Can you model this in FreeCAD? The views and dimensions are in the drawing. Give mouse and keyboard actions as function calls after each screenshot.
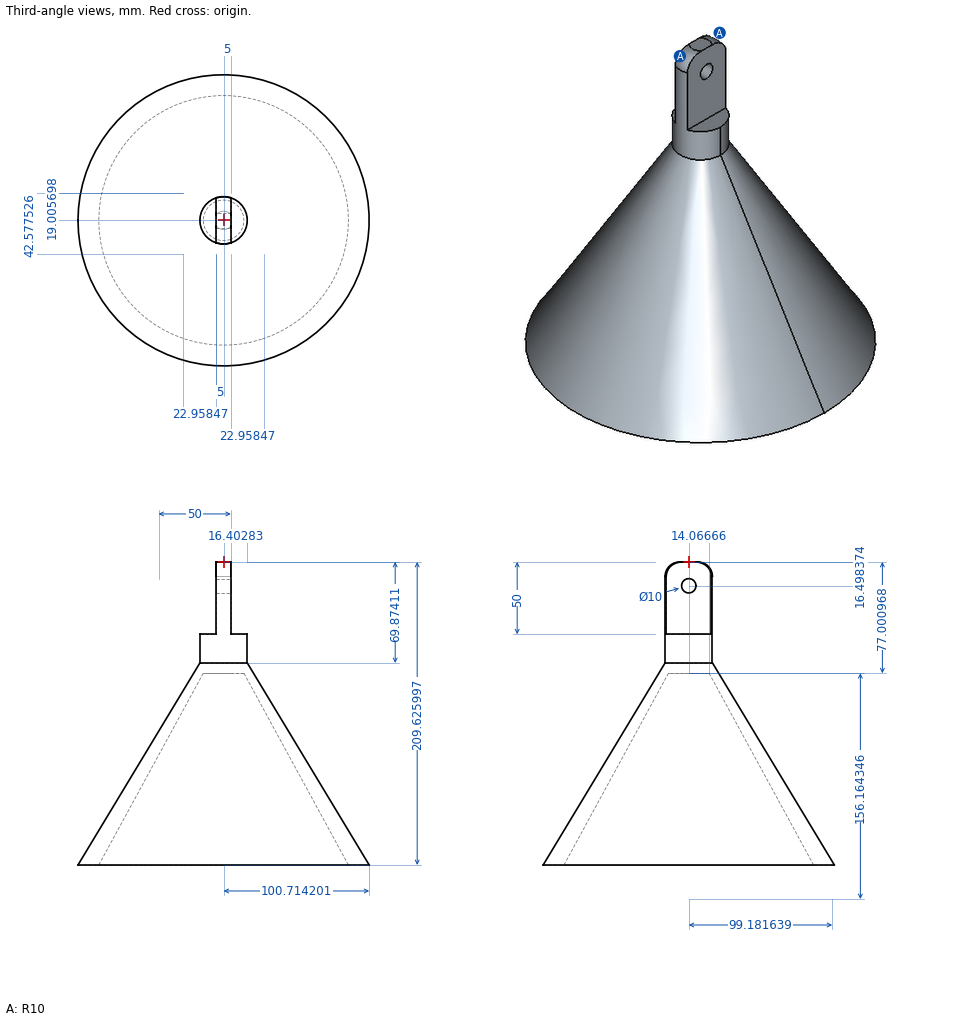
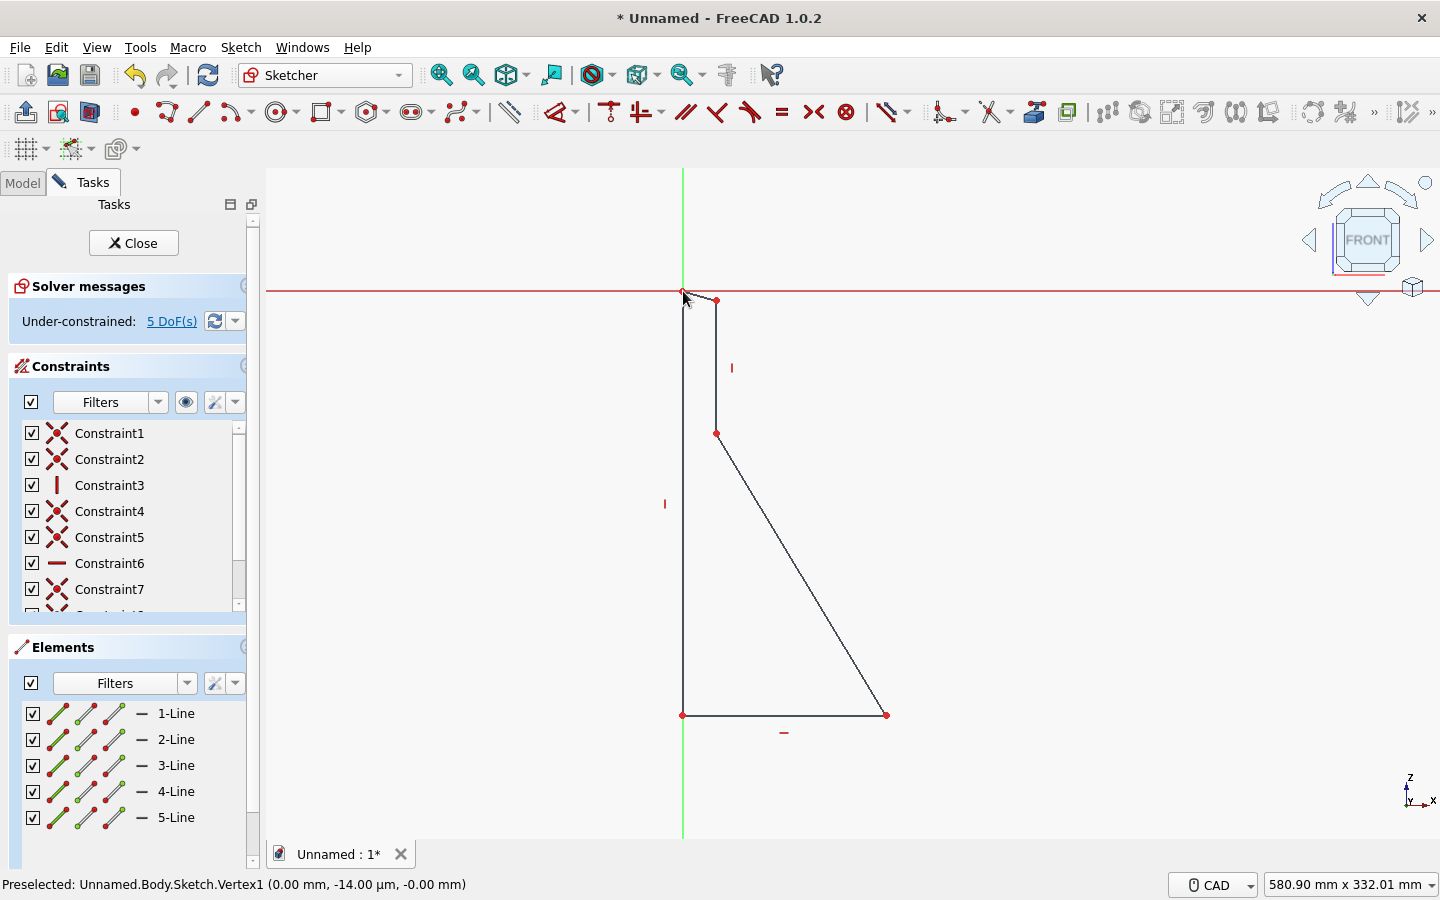
scroll(693, 294, up, 2)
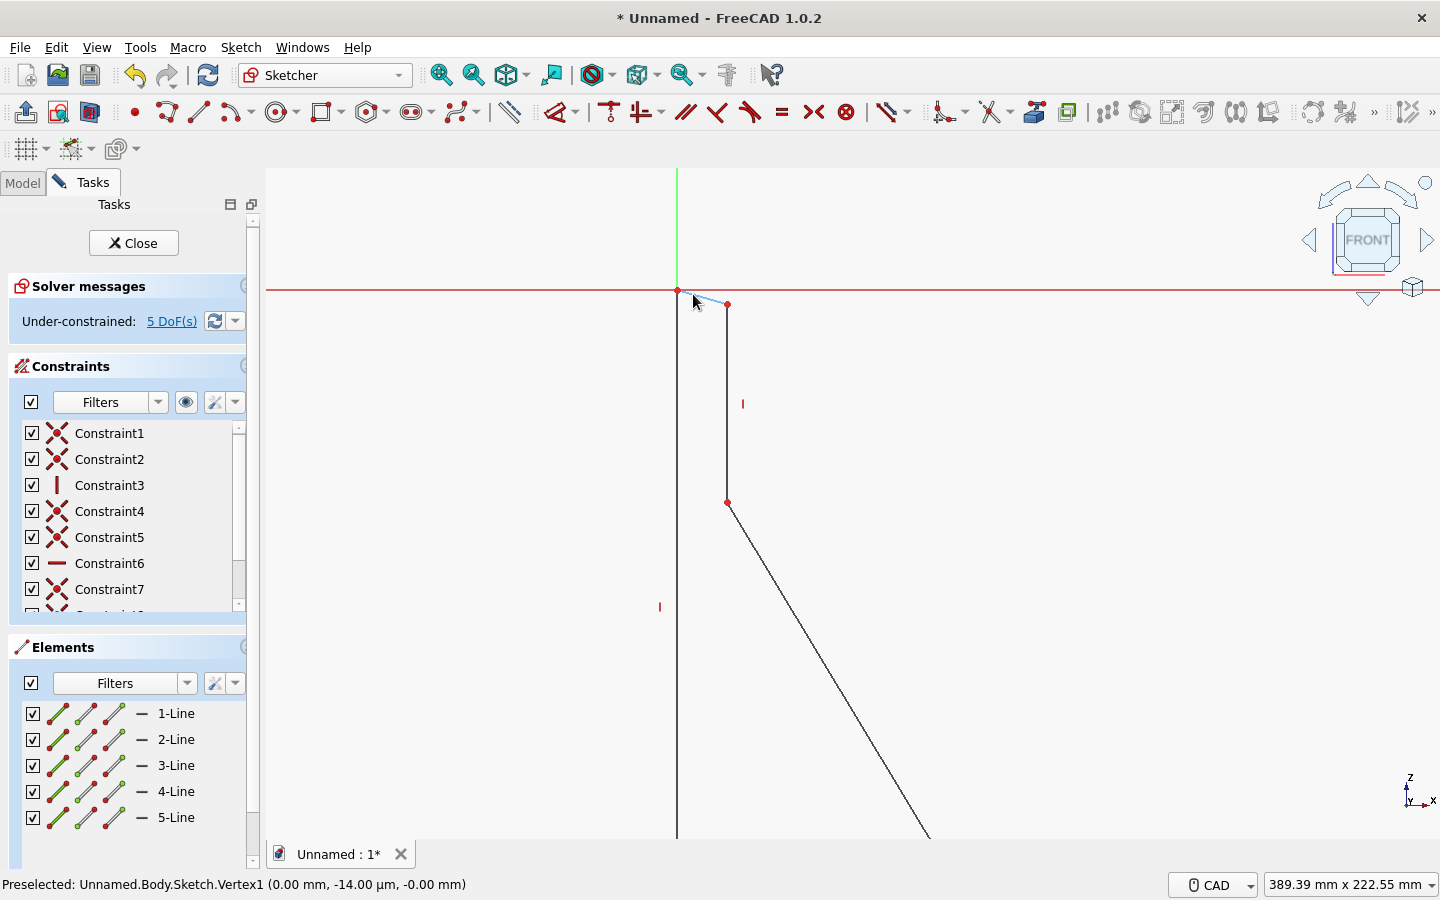
click(692, 294)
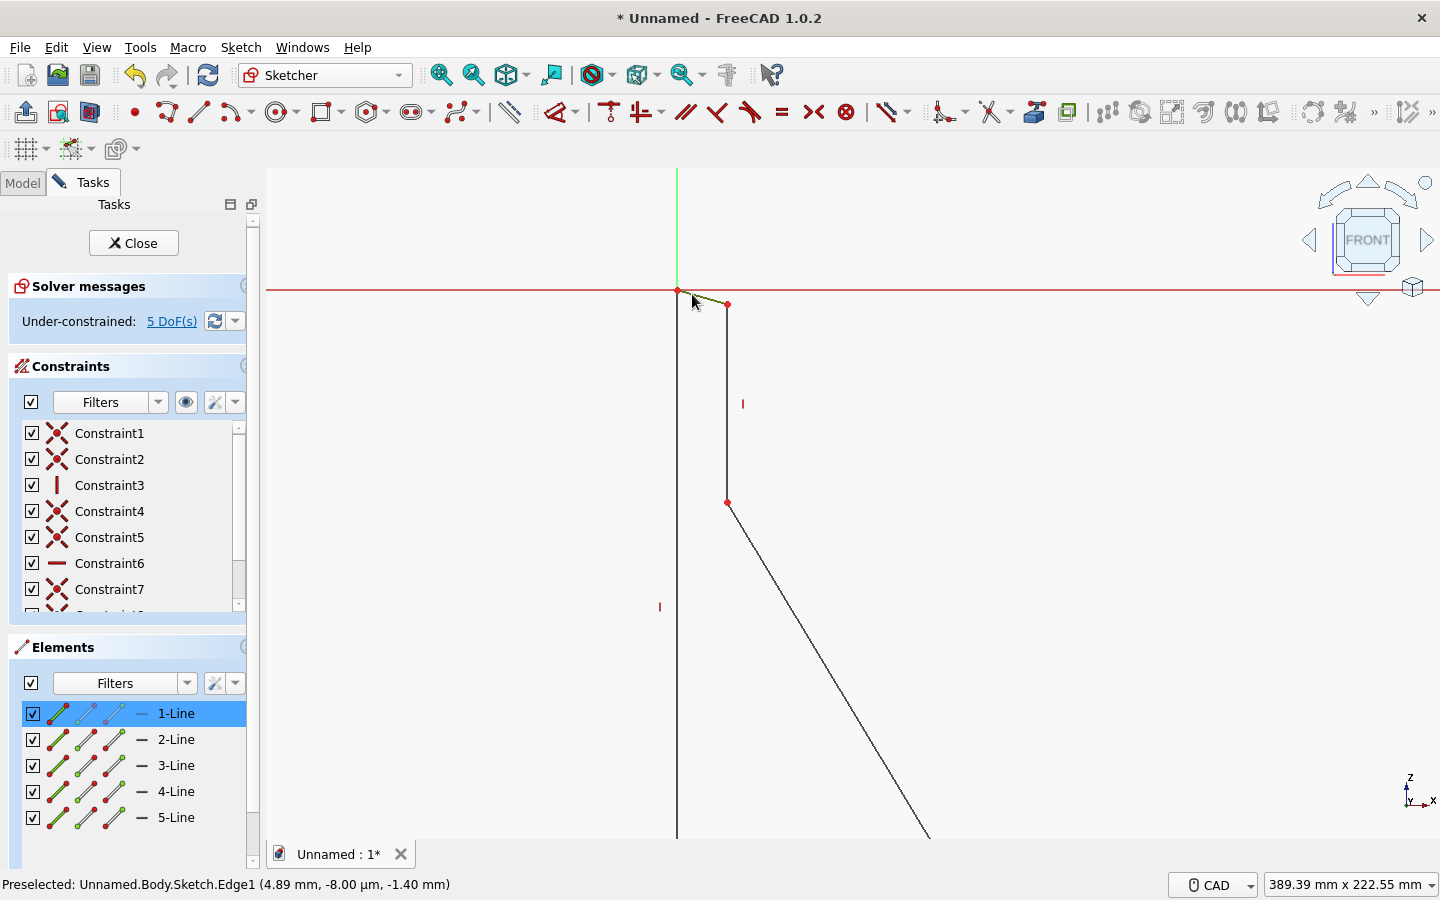
click(664, 112)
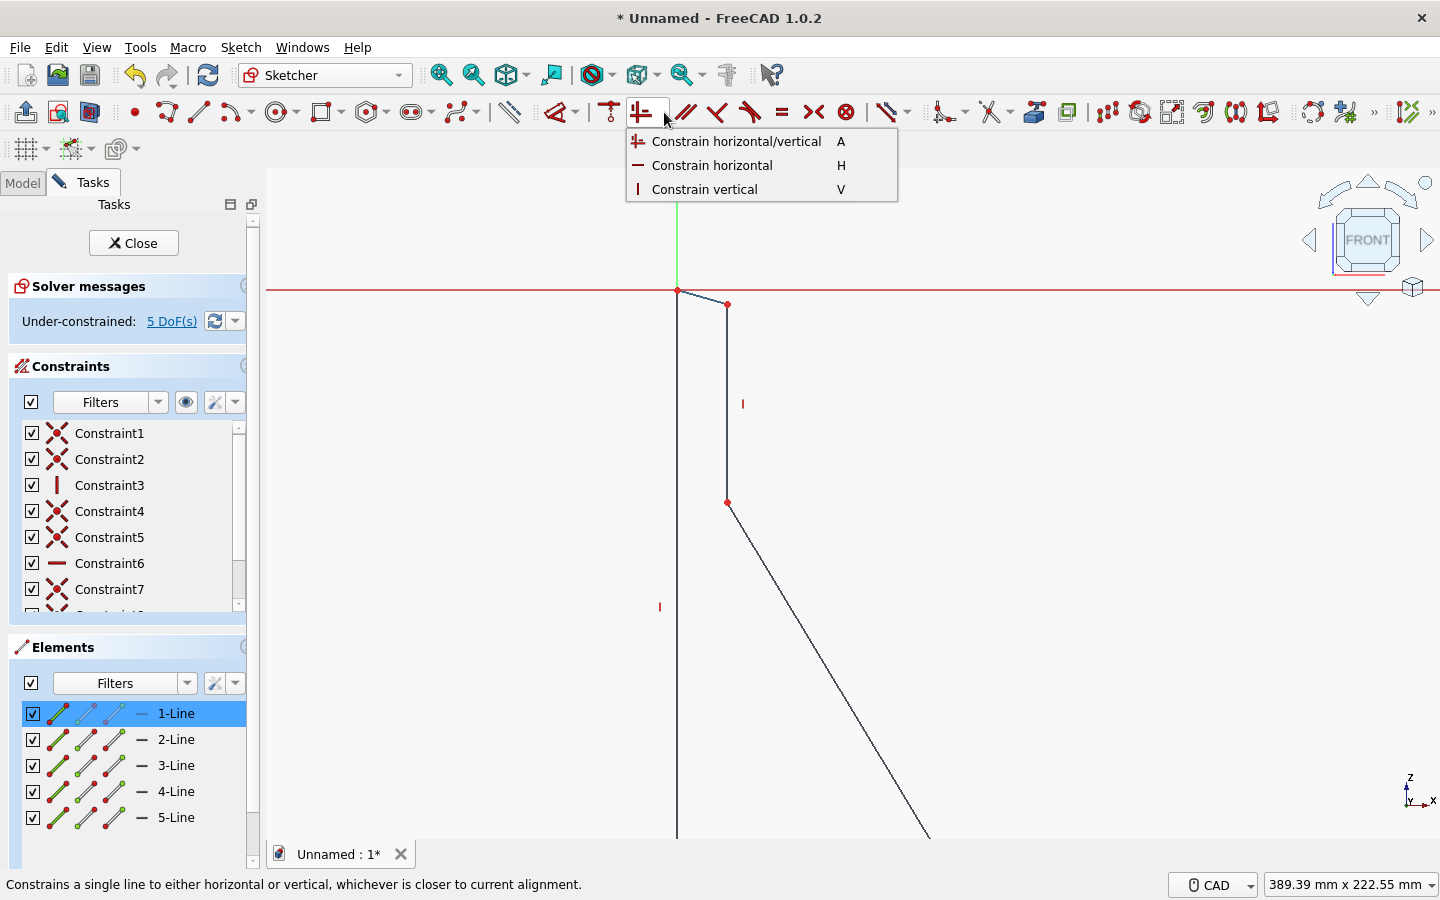
click(762, 165)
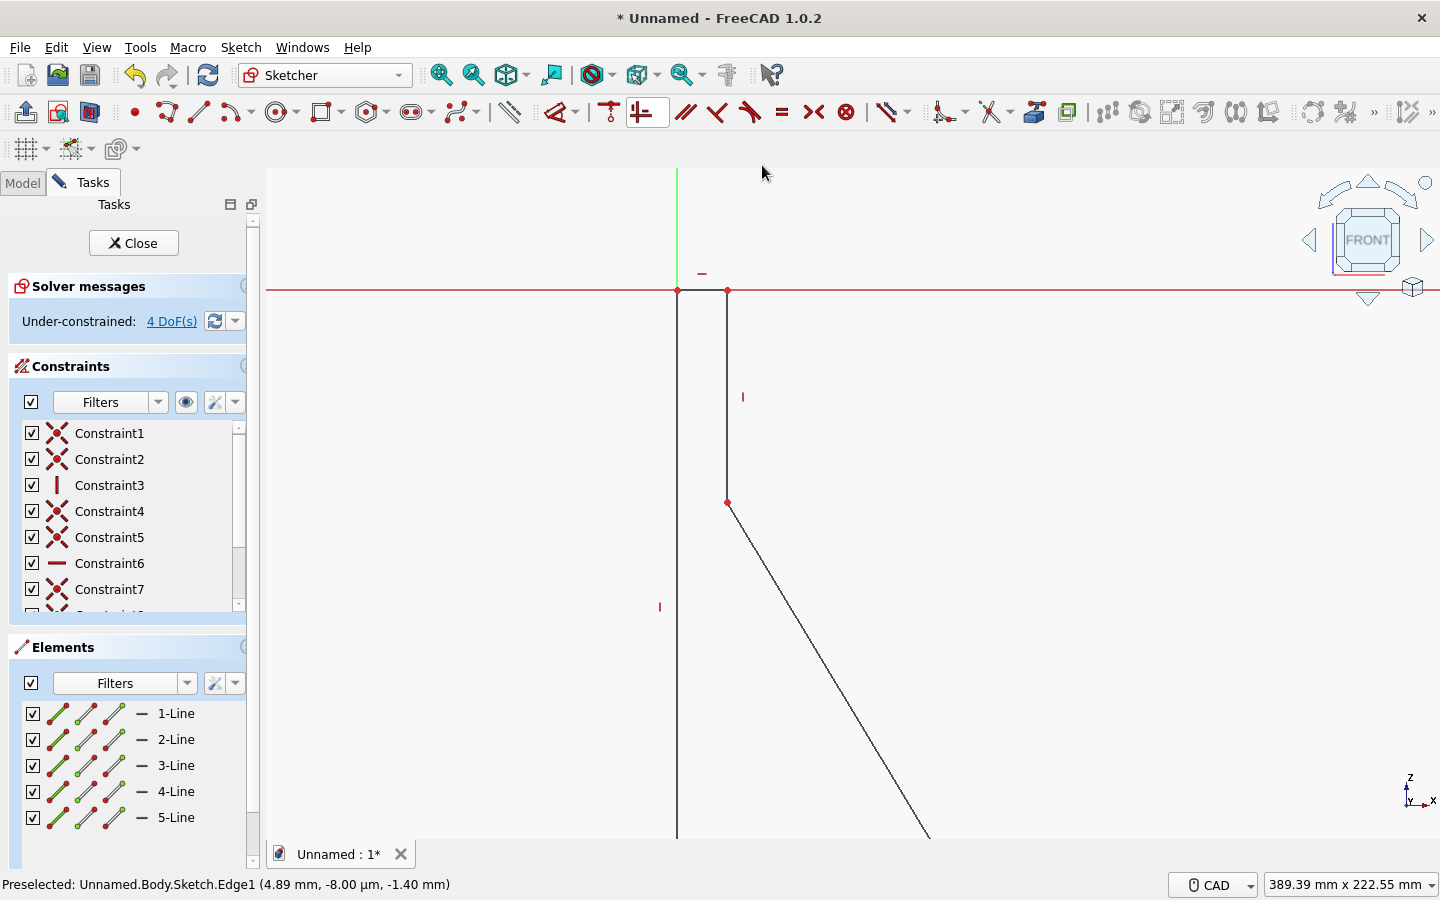
key(d)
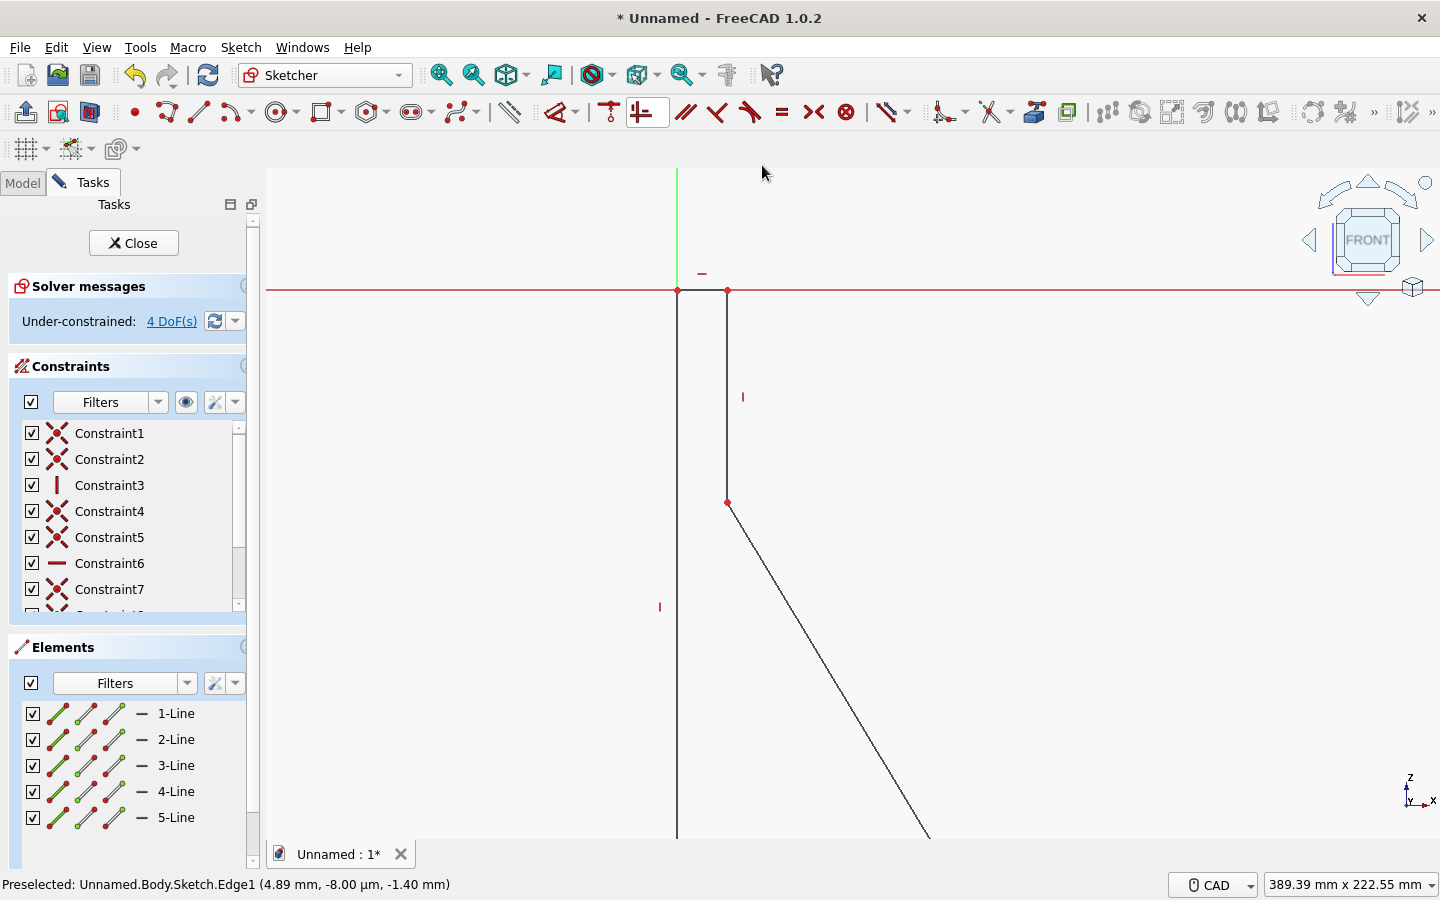
click(692, 290)
click(702, 256)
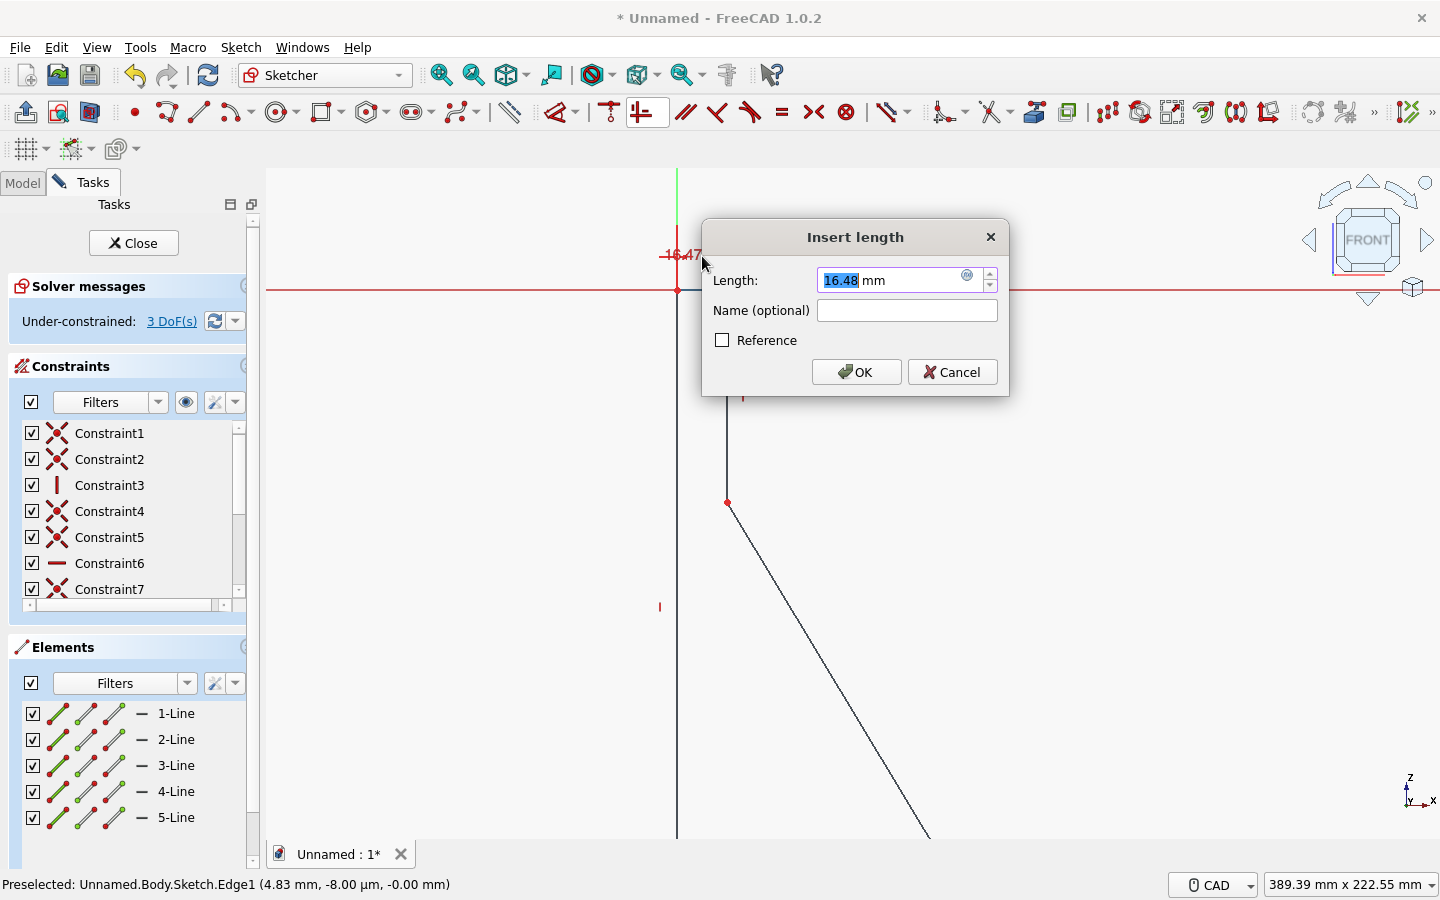
text(16.40283)
key(Return)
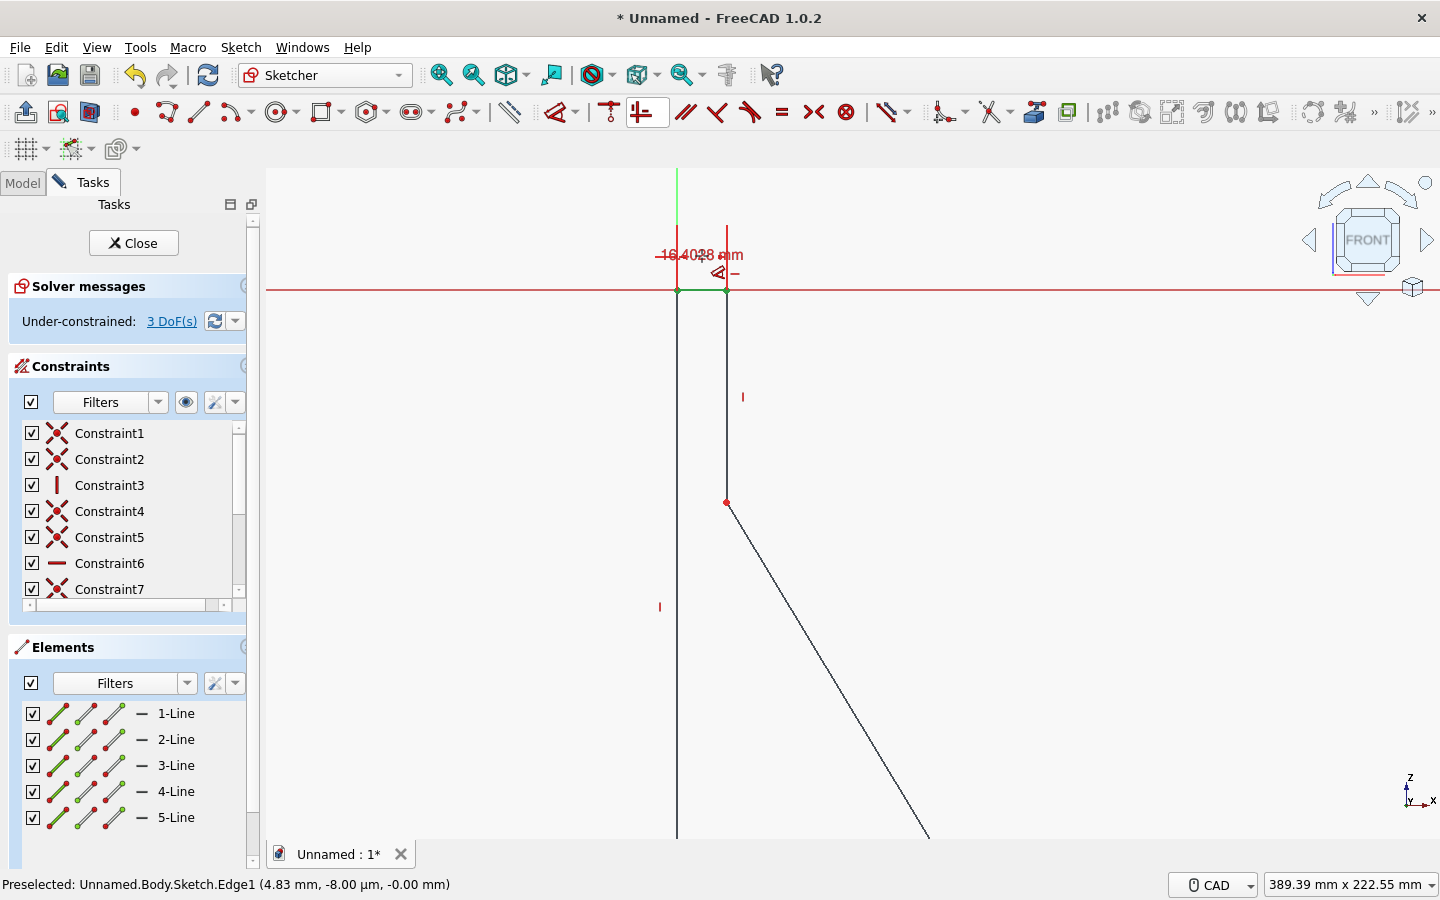
click(727, 354)
click(693, 396)